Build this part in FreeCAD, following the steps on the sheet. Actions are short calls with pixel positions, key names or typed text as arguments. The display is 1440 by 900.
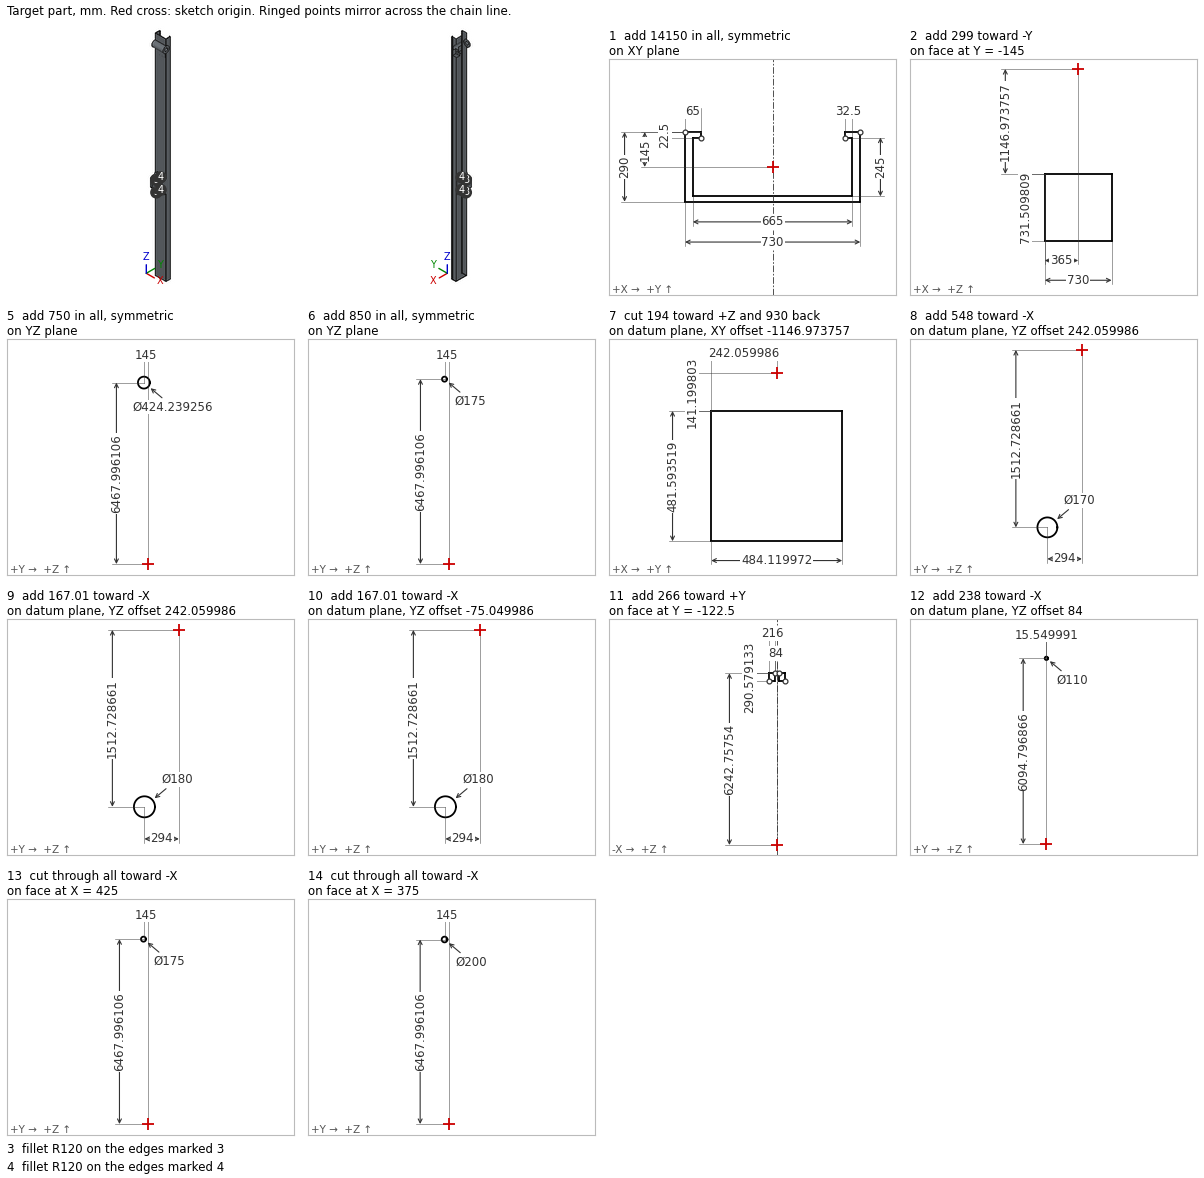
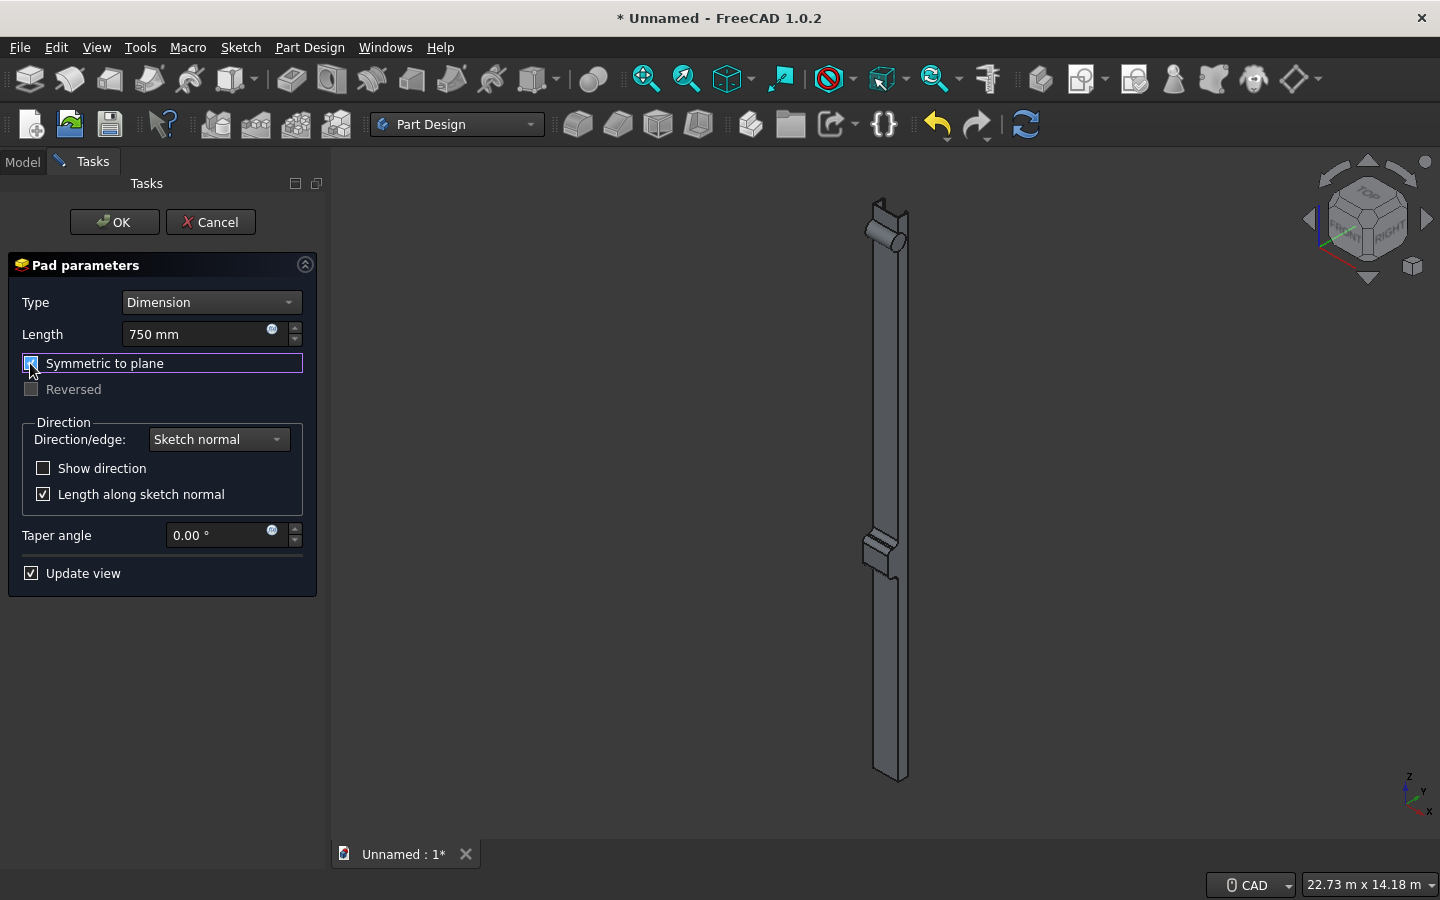
click(115, 222)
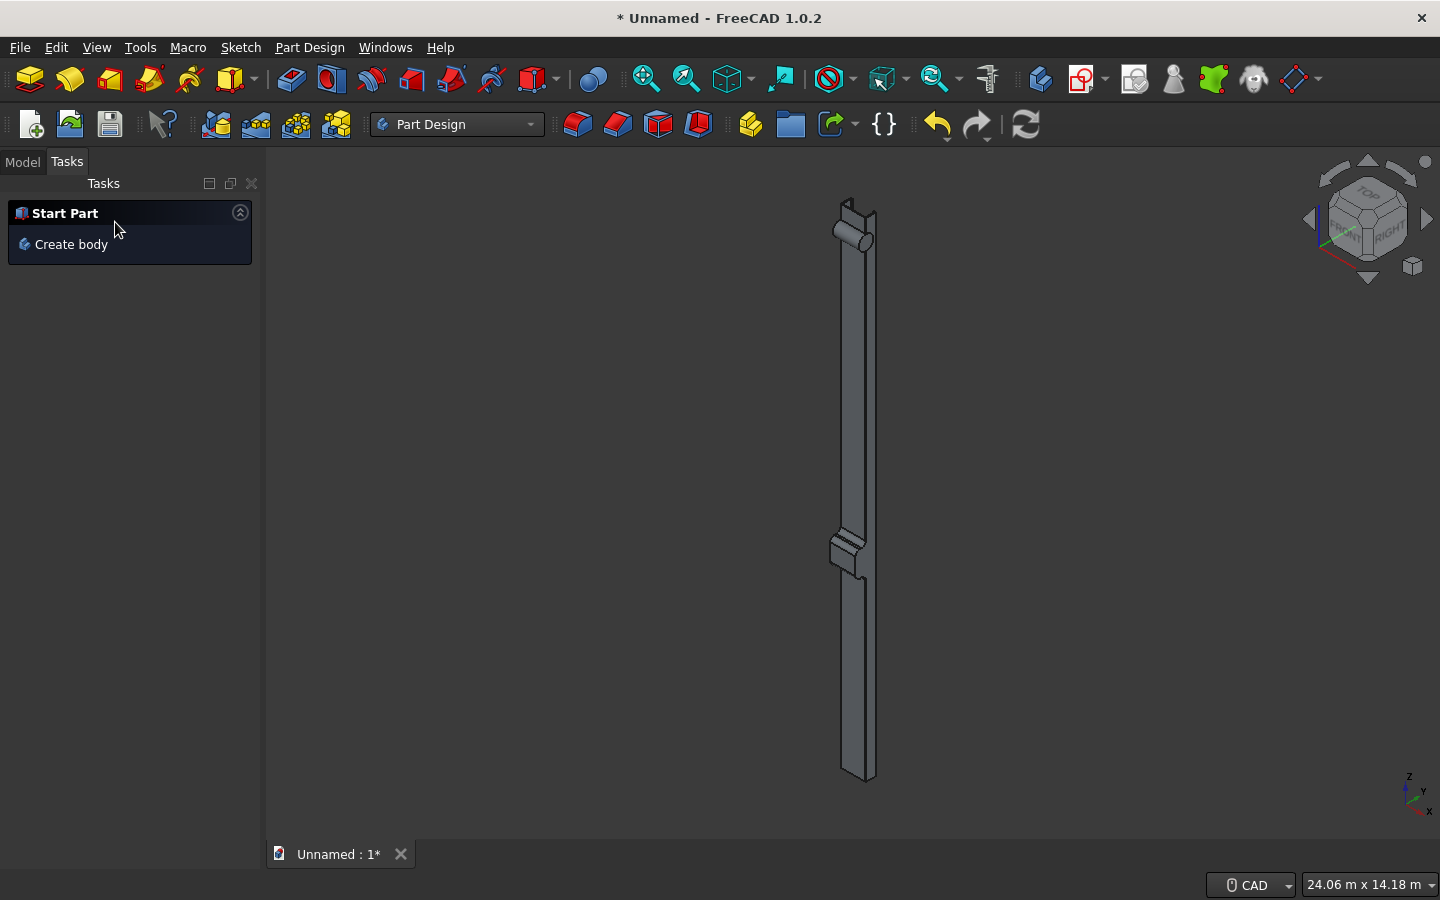
click(1082, 80)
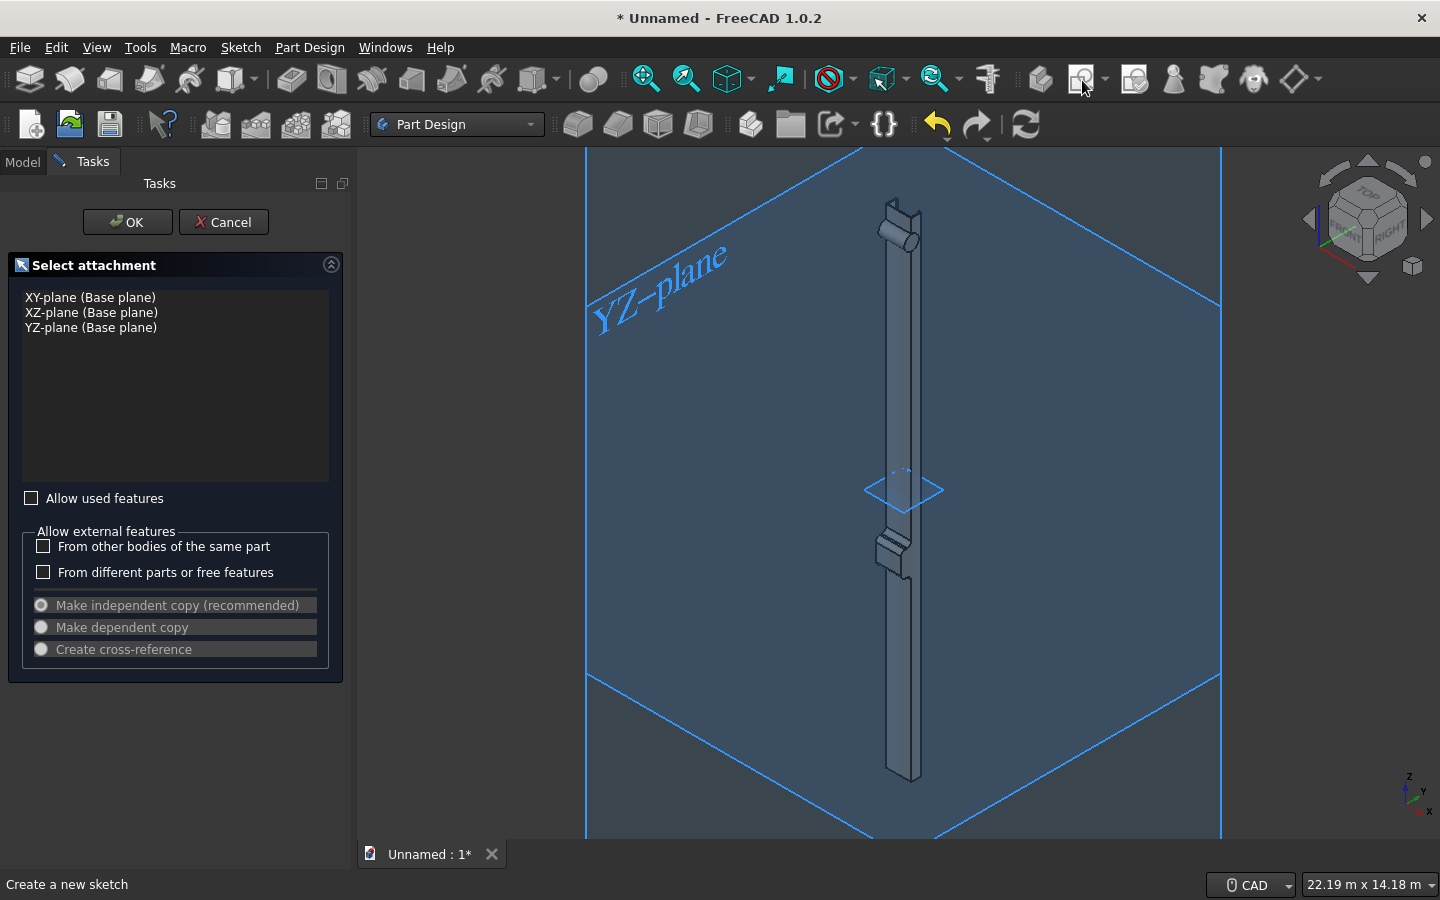
click(82, 328)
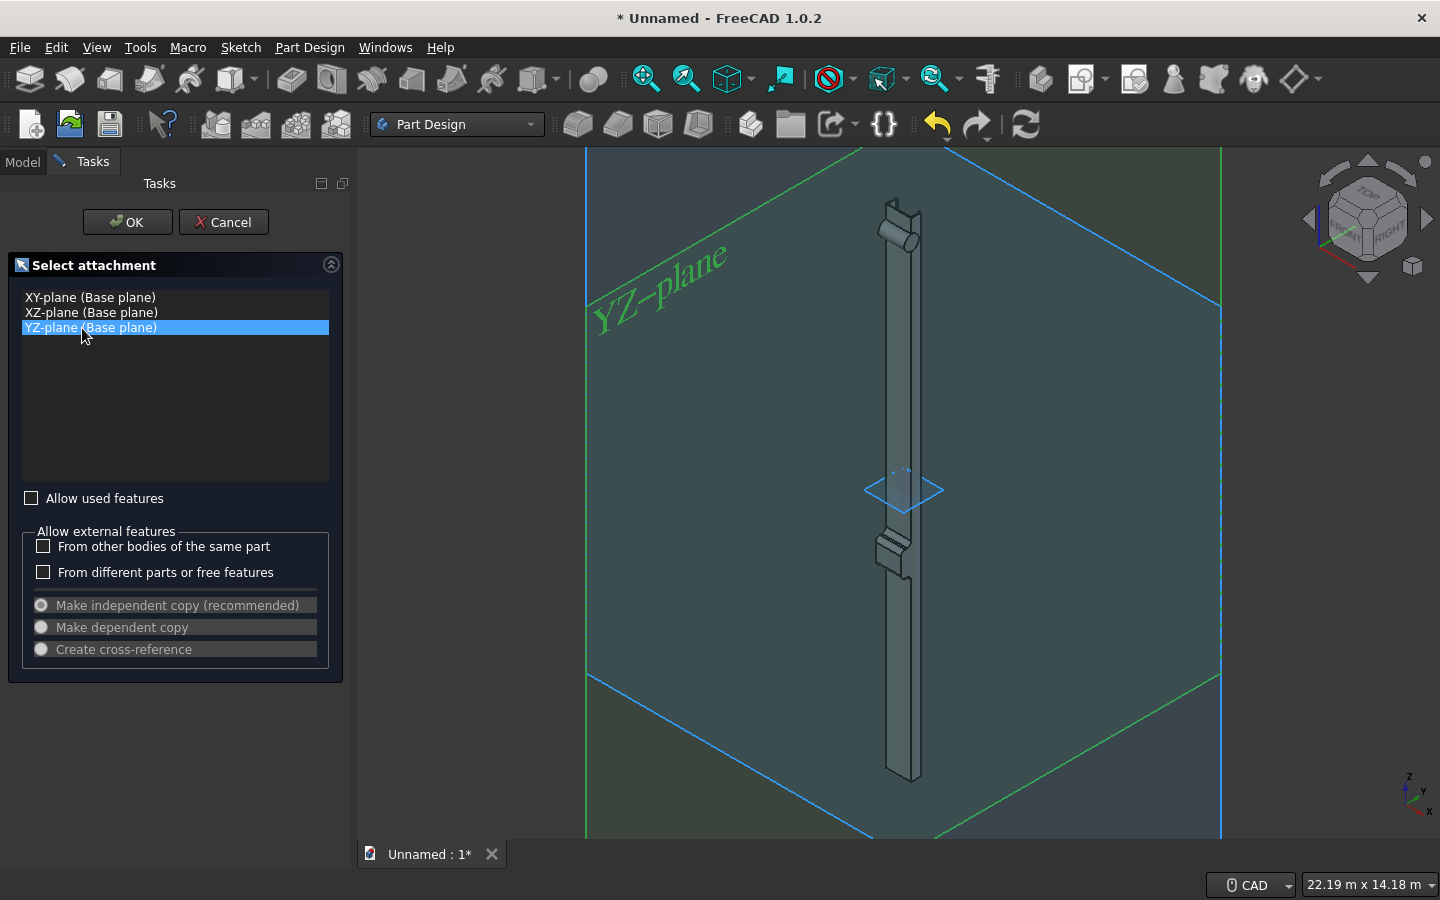
click(128, 222)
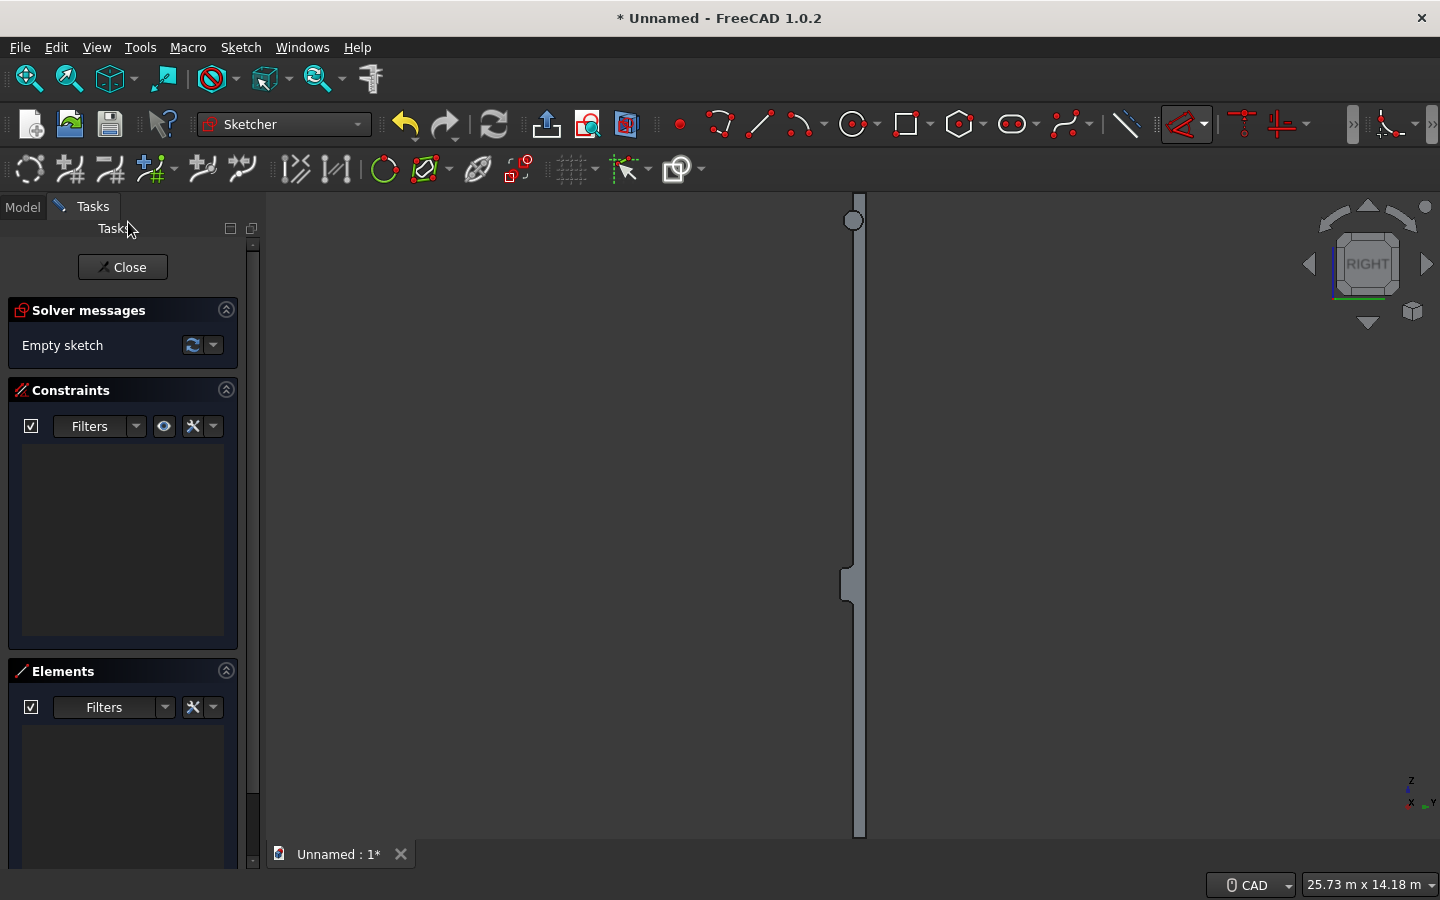
key(q)
key(s)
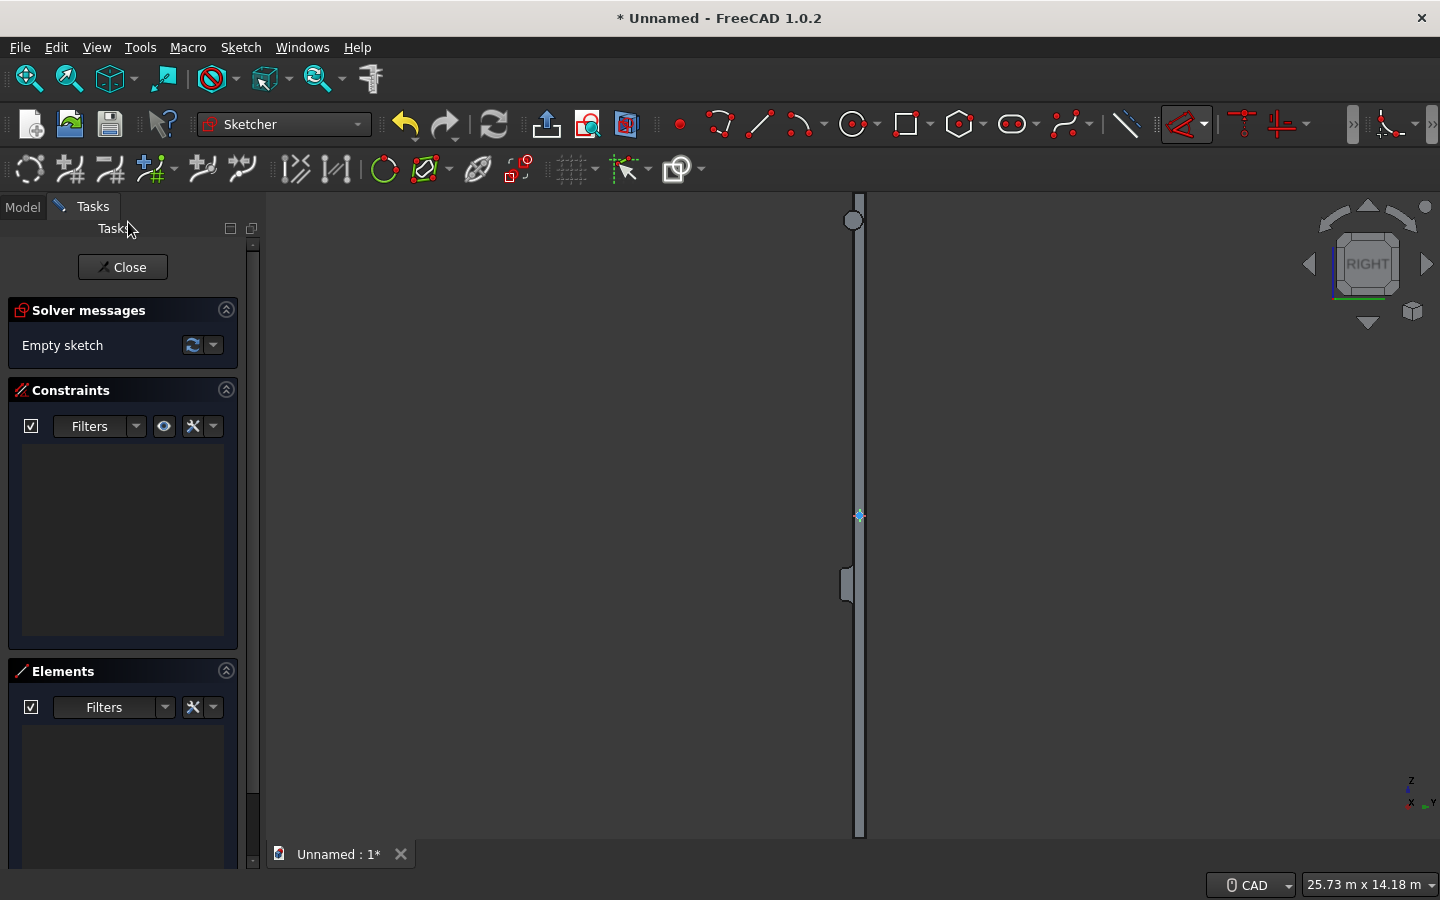
scroll(784, 516, down, 5)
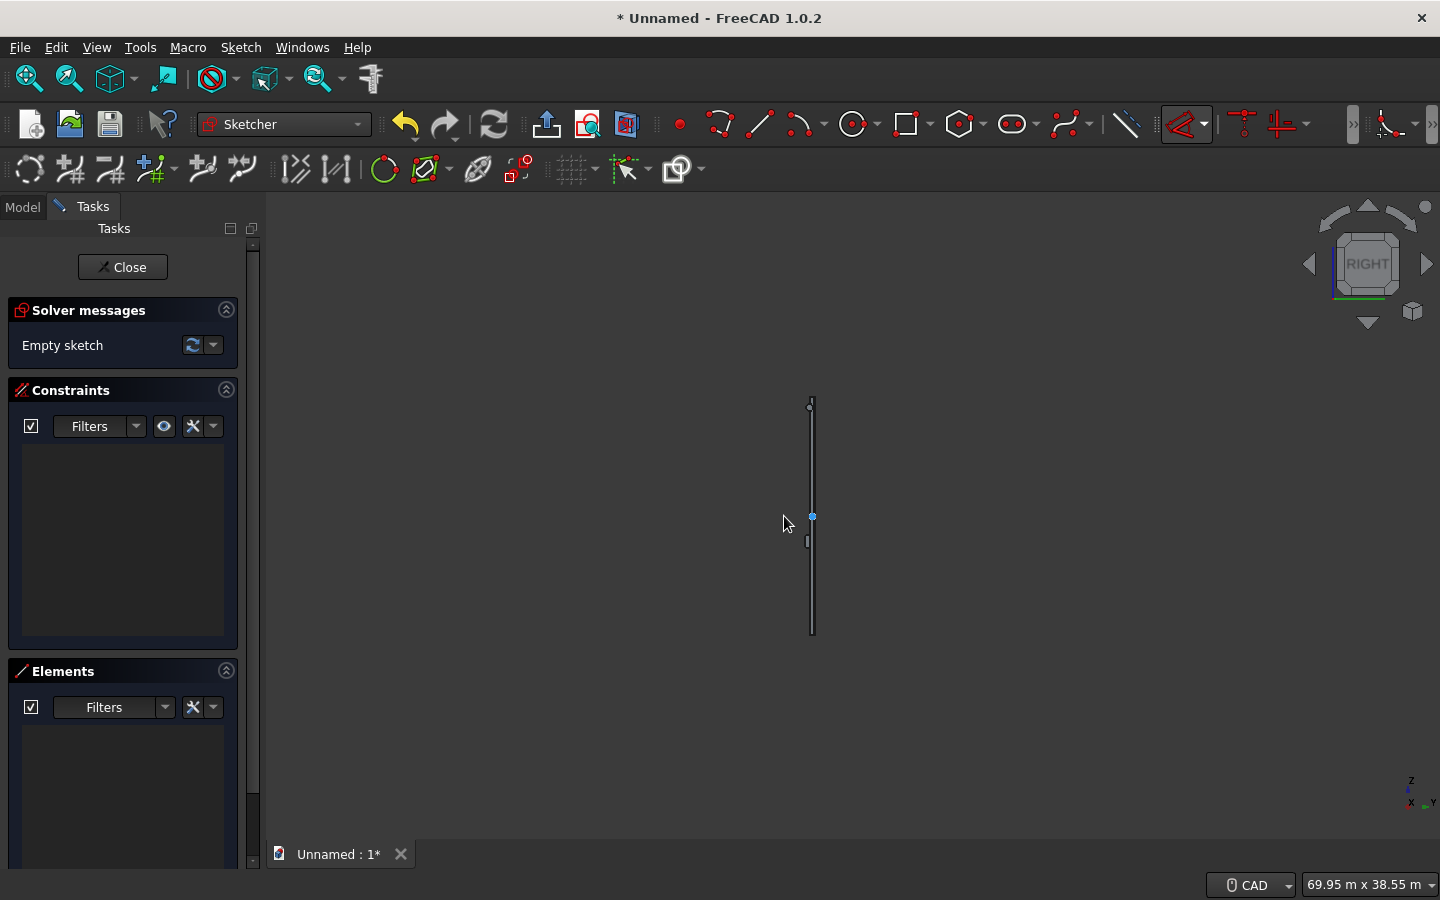
scroll(811, 402, up, 15)